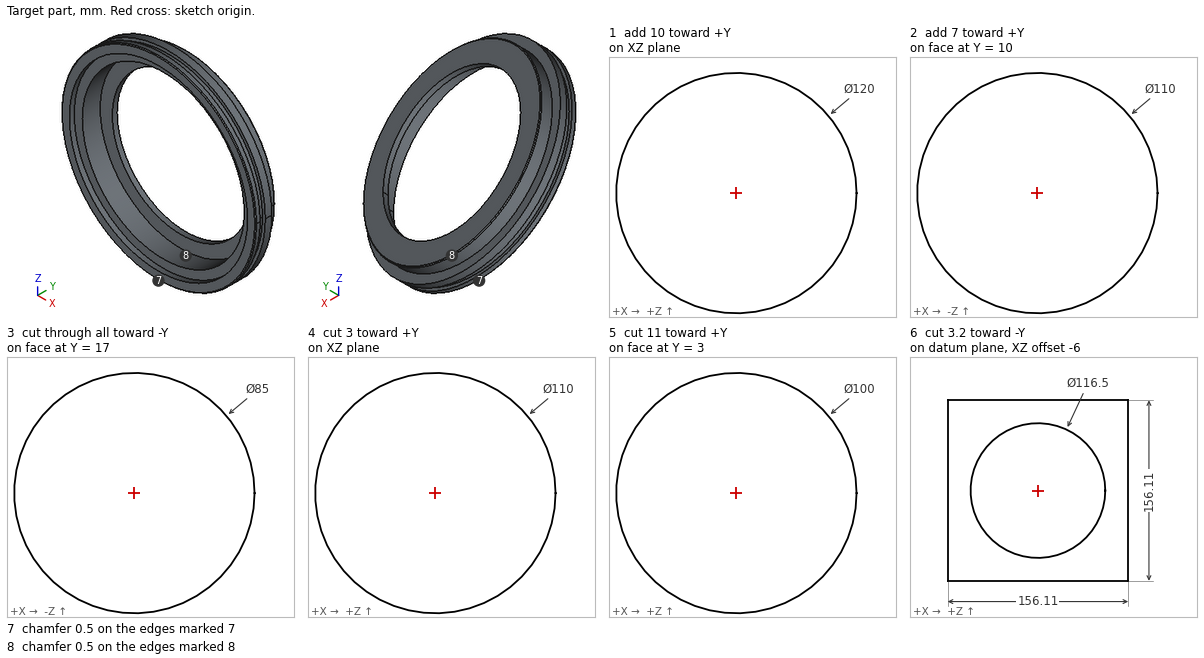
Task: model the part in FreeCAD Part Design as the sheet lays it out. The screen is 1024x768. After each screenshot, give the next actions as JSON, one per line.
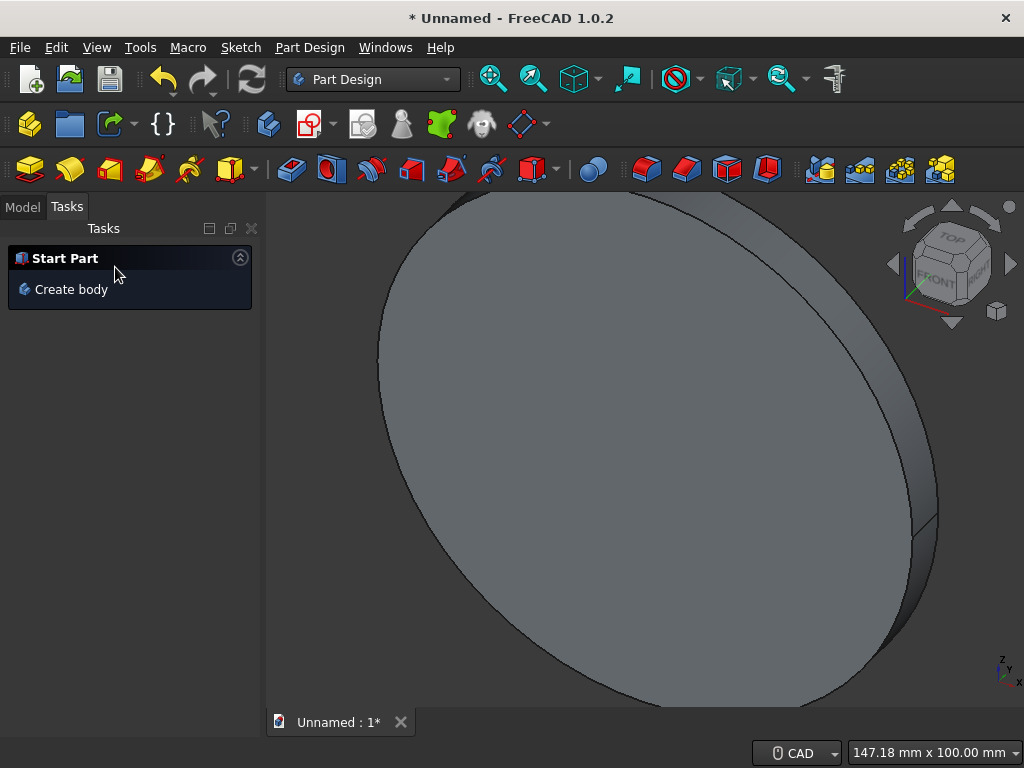
{"action": "key", "text": "v f"}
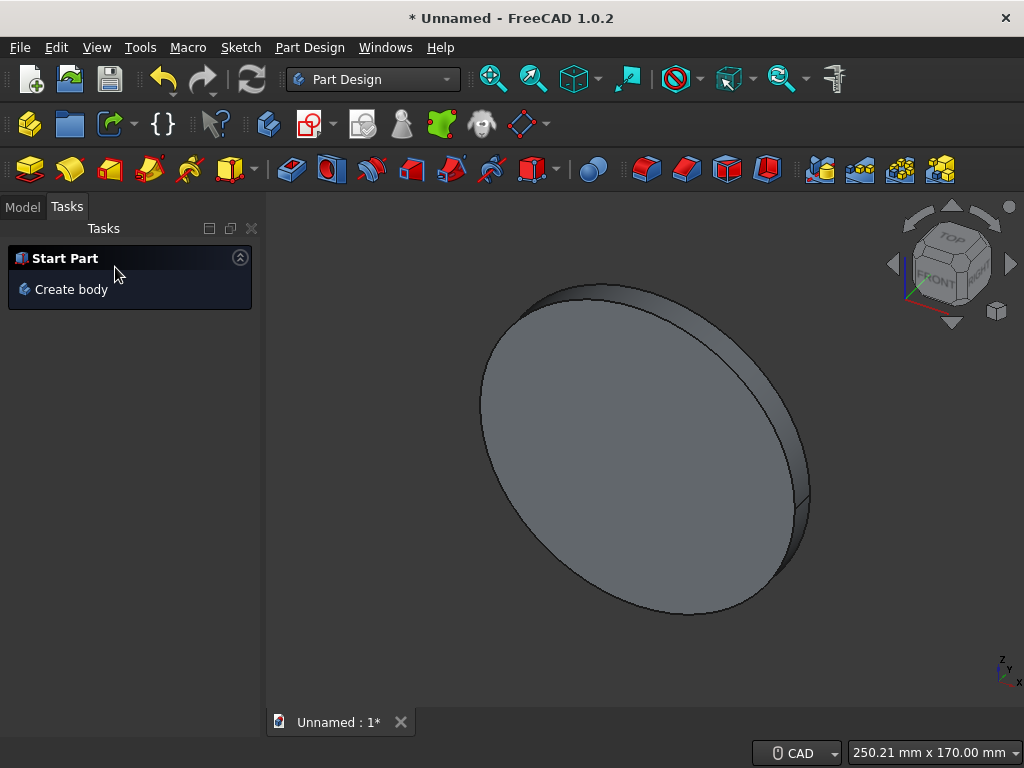
{"action": "key", "text": "4"}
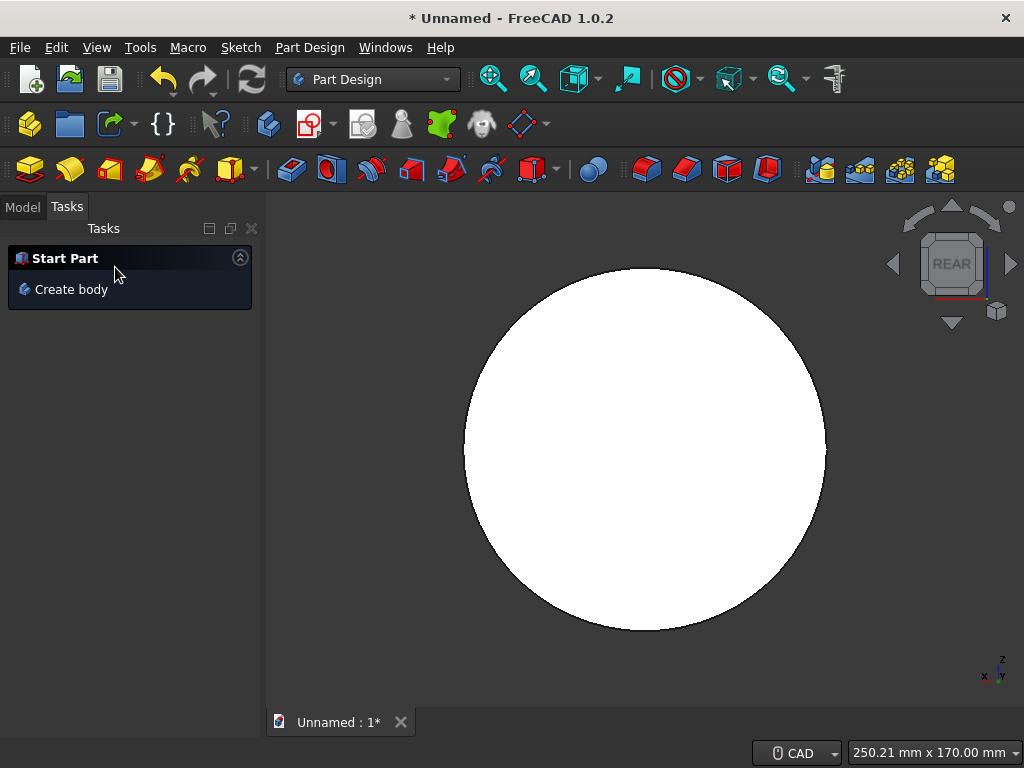
{"action": "left_click", "coordinate": [645, 448]}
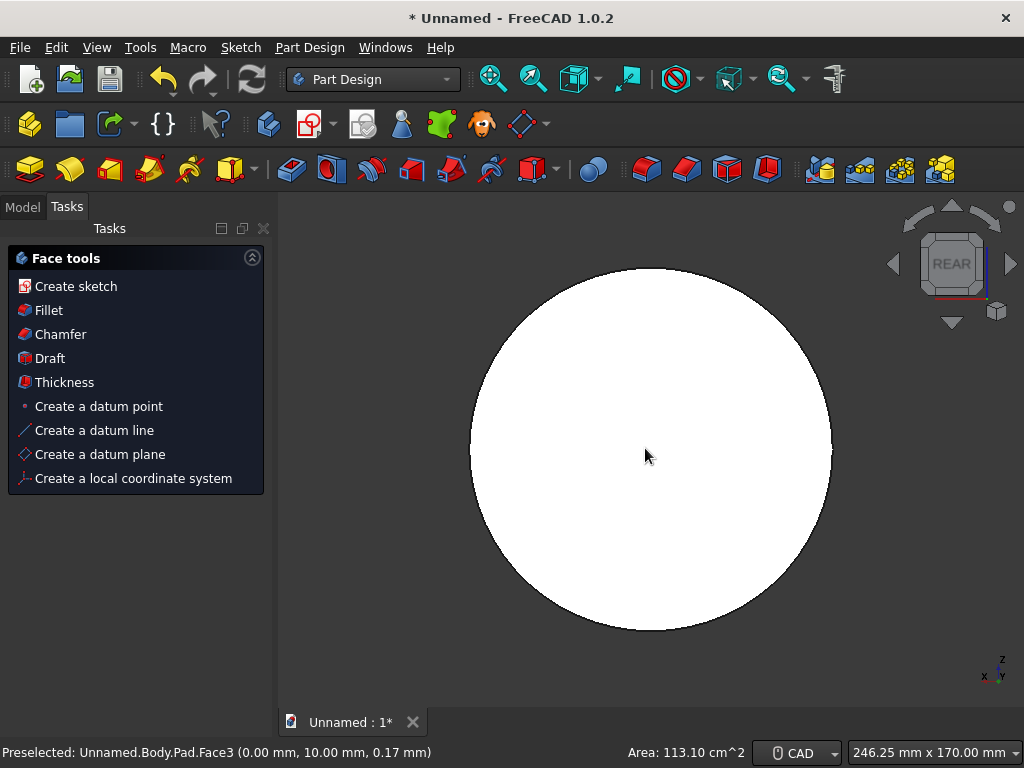
{"action": "left_click", "coordinate": [310, 124]}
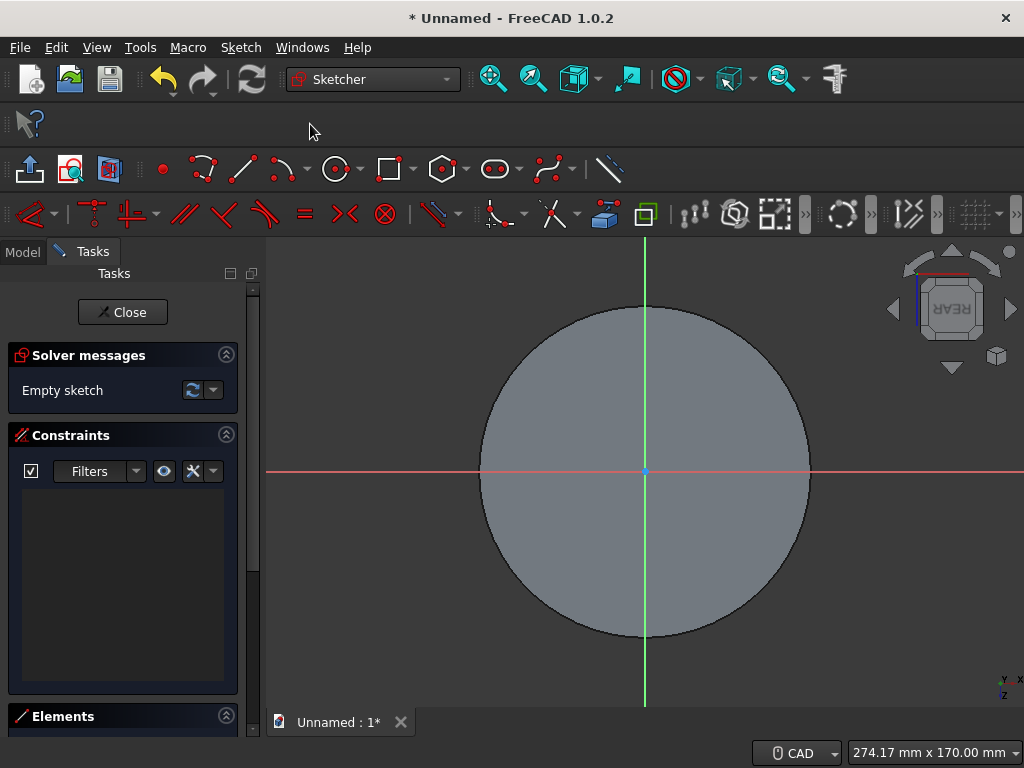
{"action": "left_click", "coordinate": [336, 170]}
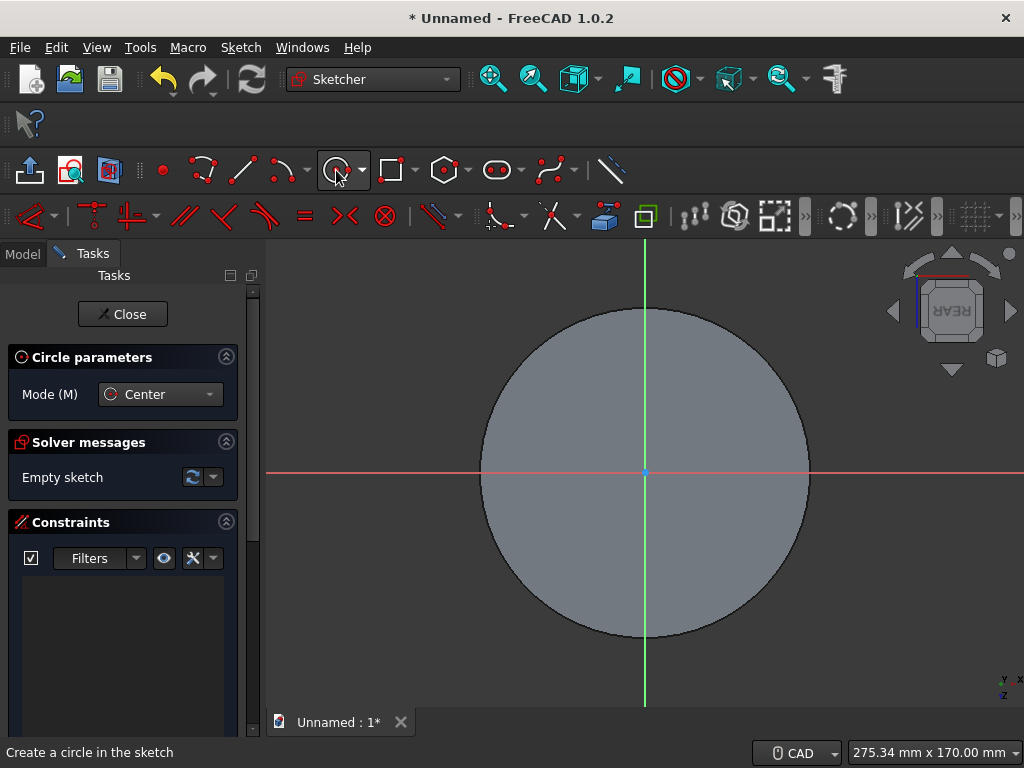
{"action": "left_click", "coordinate": [645, 473]}
{"action": "mouse_move", "coordinate": [752, 366]}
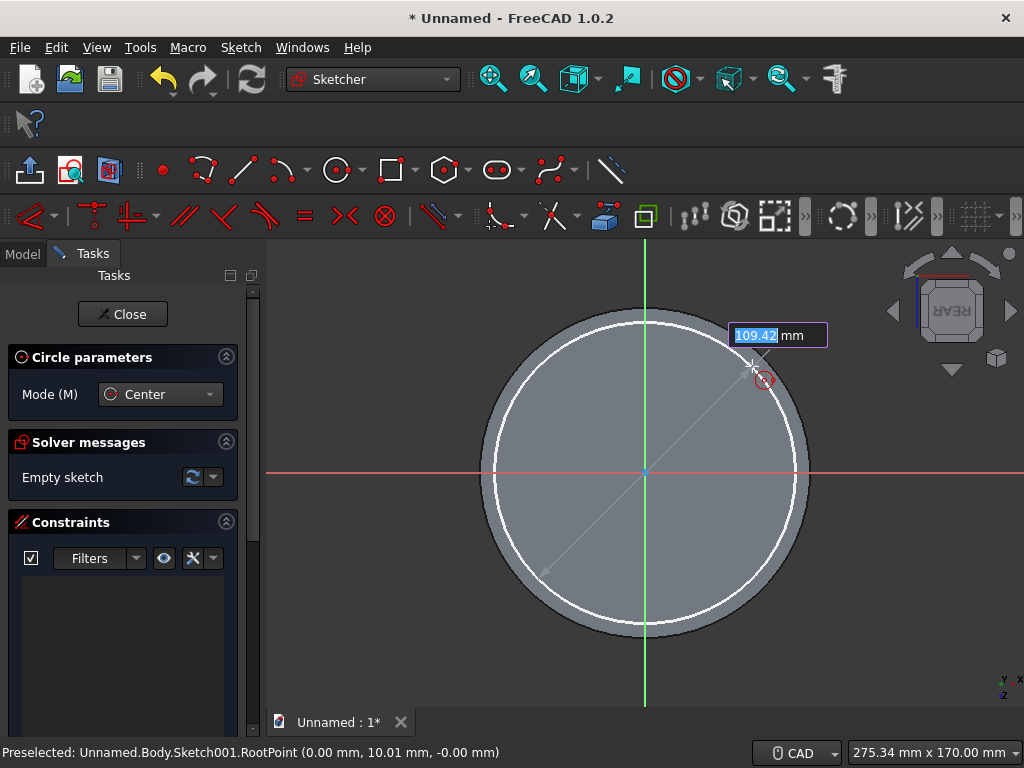
{"action": "type", "text": "110"}
{"action": "key", "text": "Return"}
{"action": "key", "text": "Escape"}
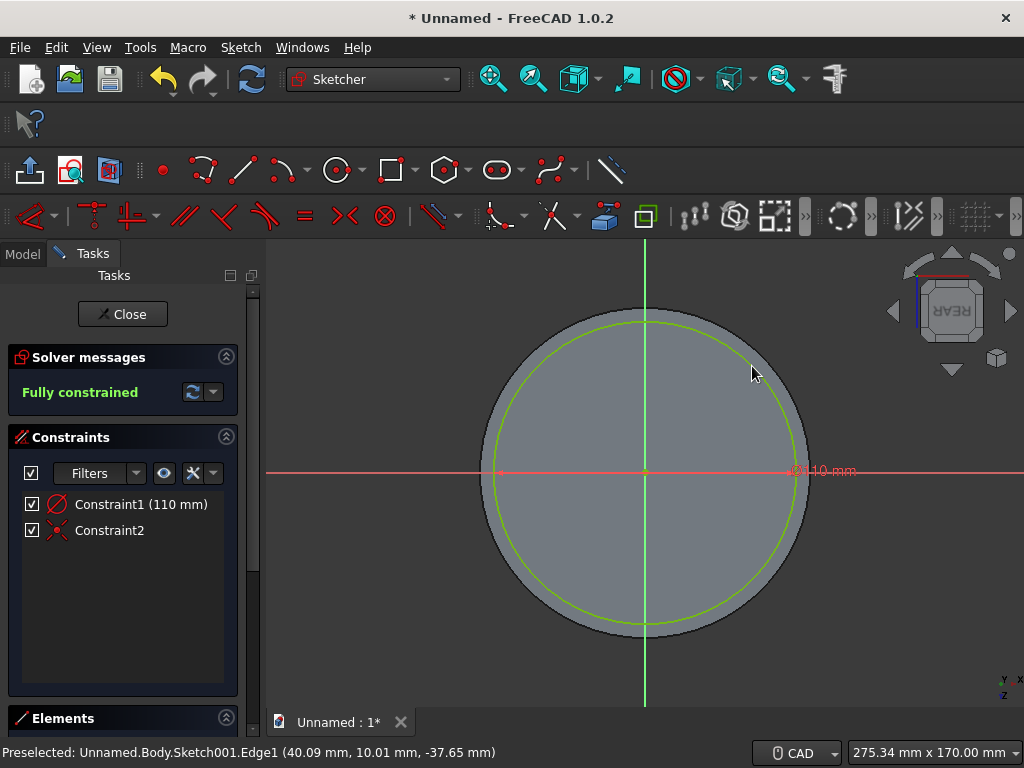
{"action": "left_click", "coordinate": [123, 314]}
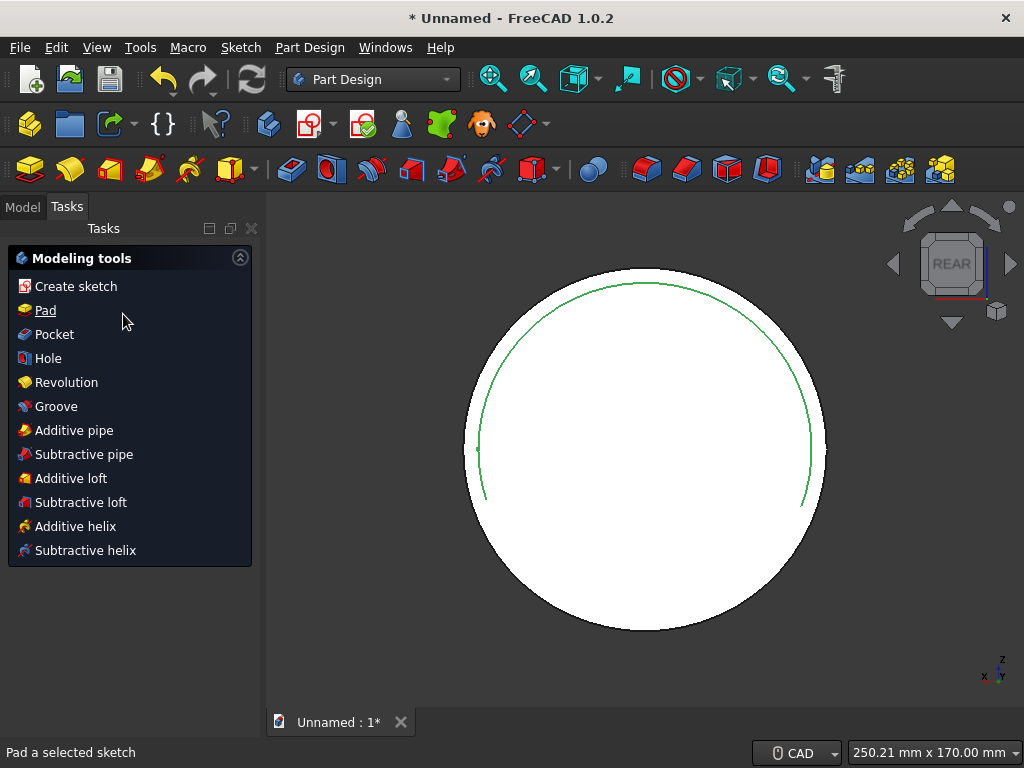
{"action": "left_click", "coordinate": [30, 170]}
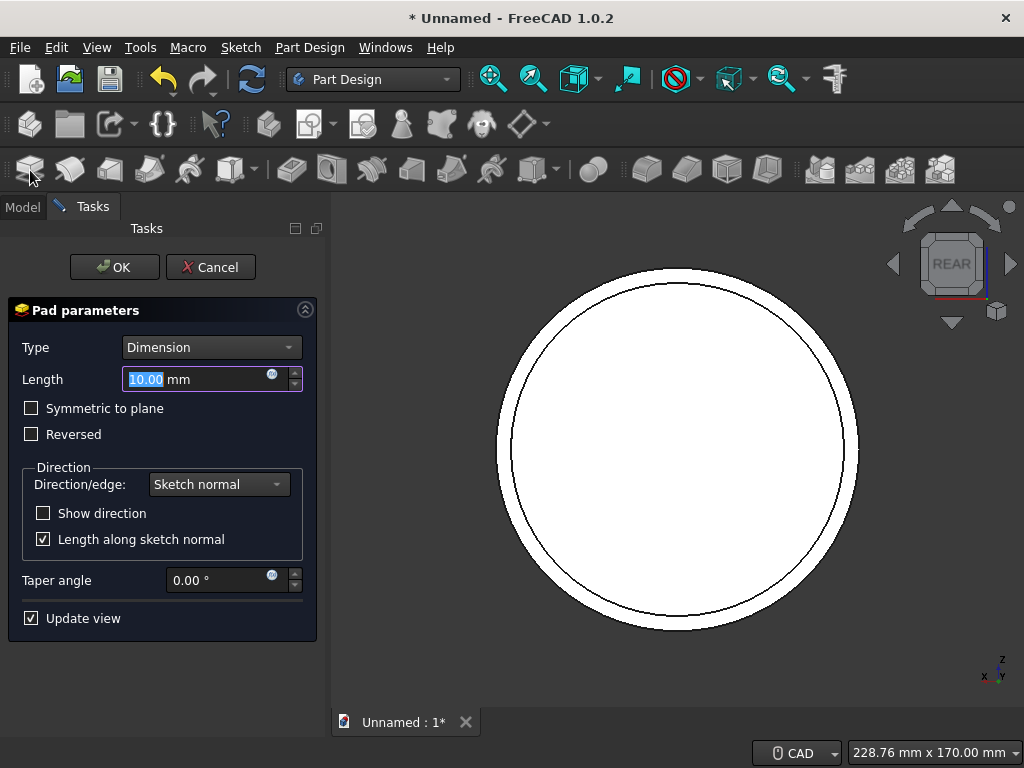
{"action": "type", "text": "7"}
{"action": "key", "text": "Tab"}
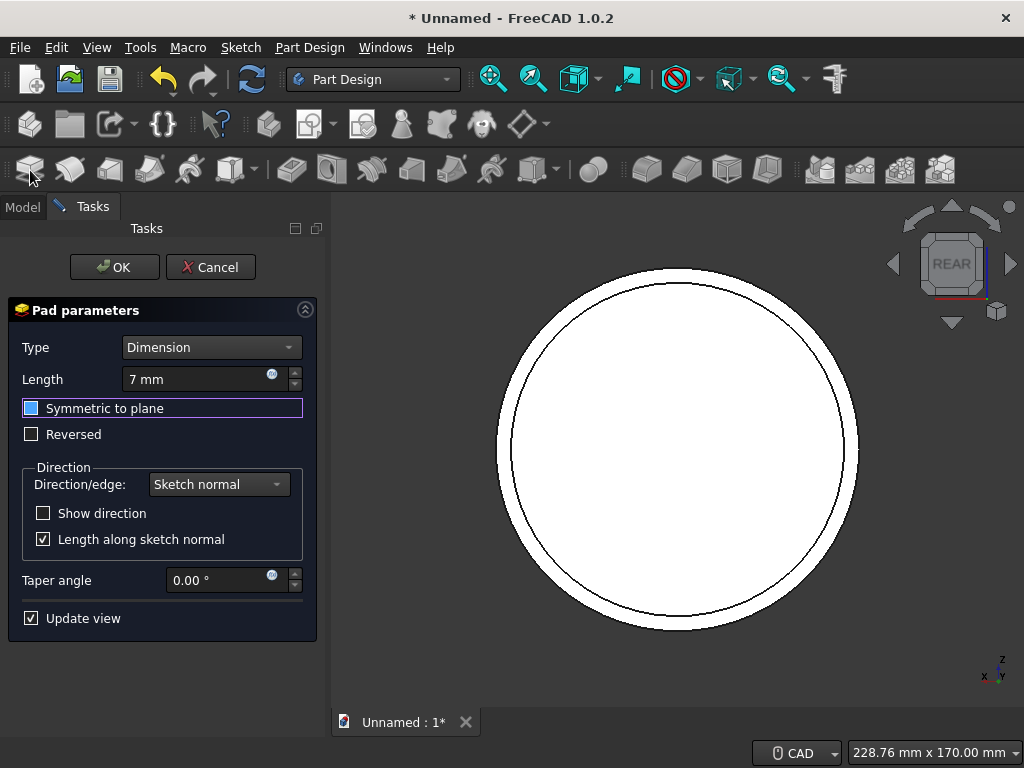
{"action": "left_click", "coordinate": [115, 267]}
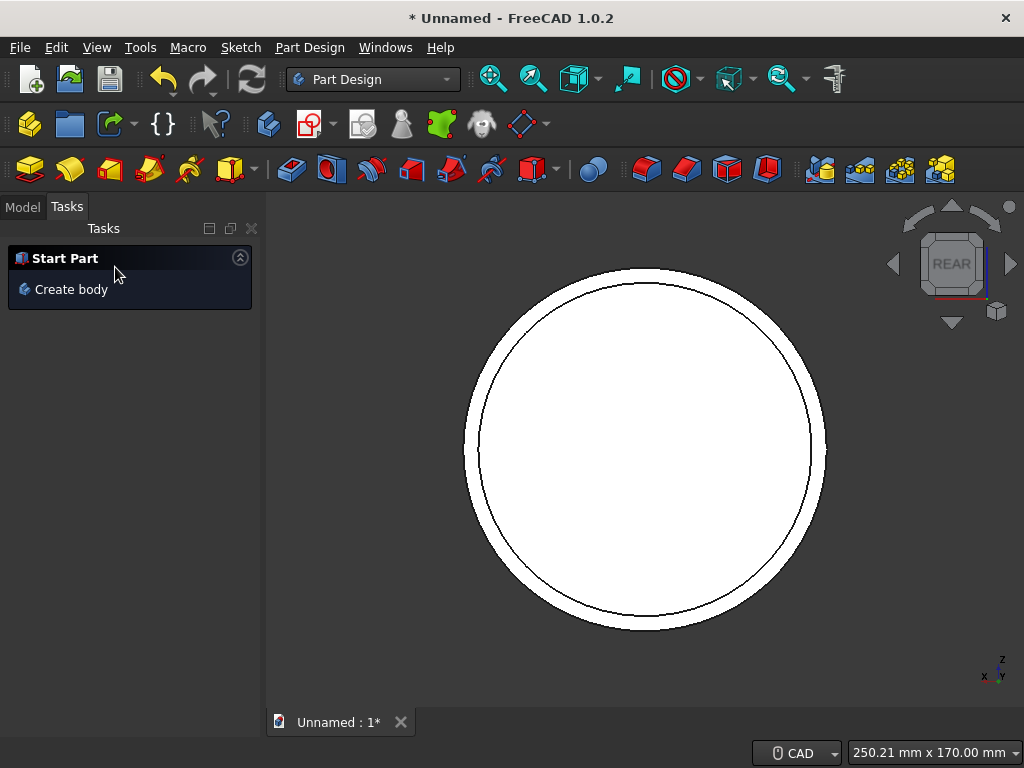
{"action": "left_click", "coordinate": [645, 448]}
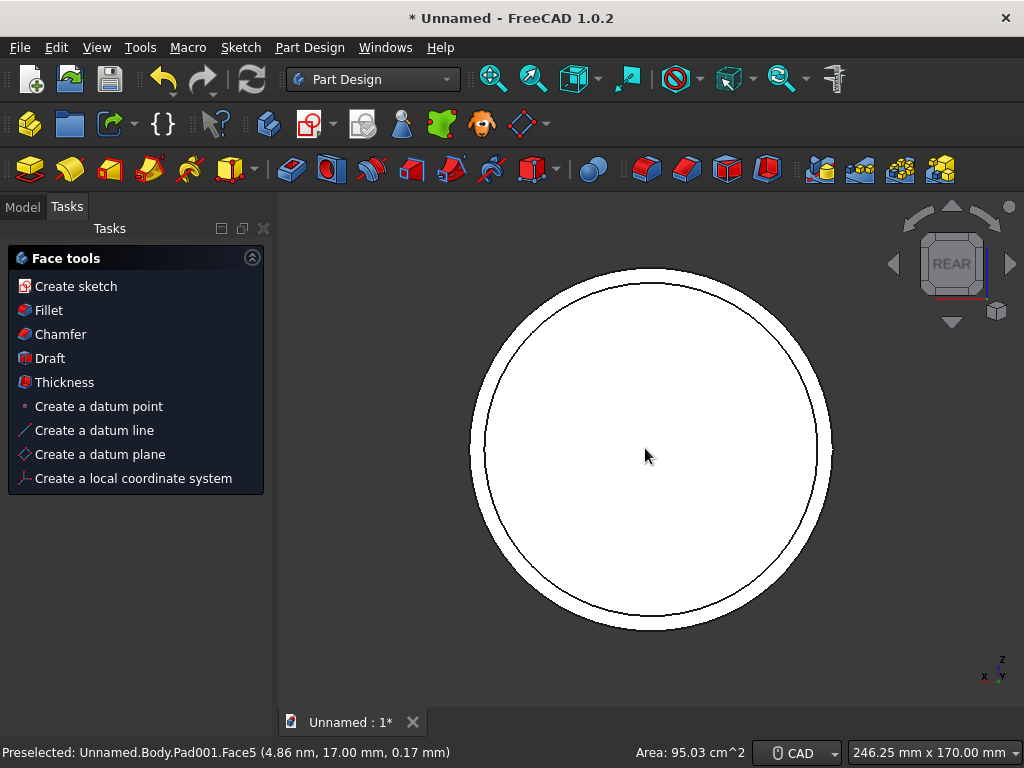
{"action": "left_click", "coordinate": [310, 124]}